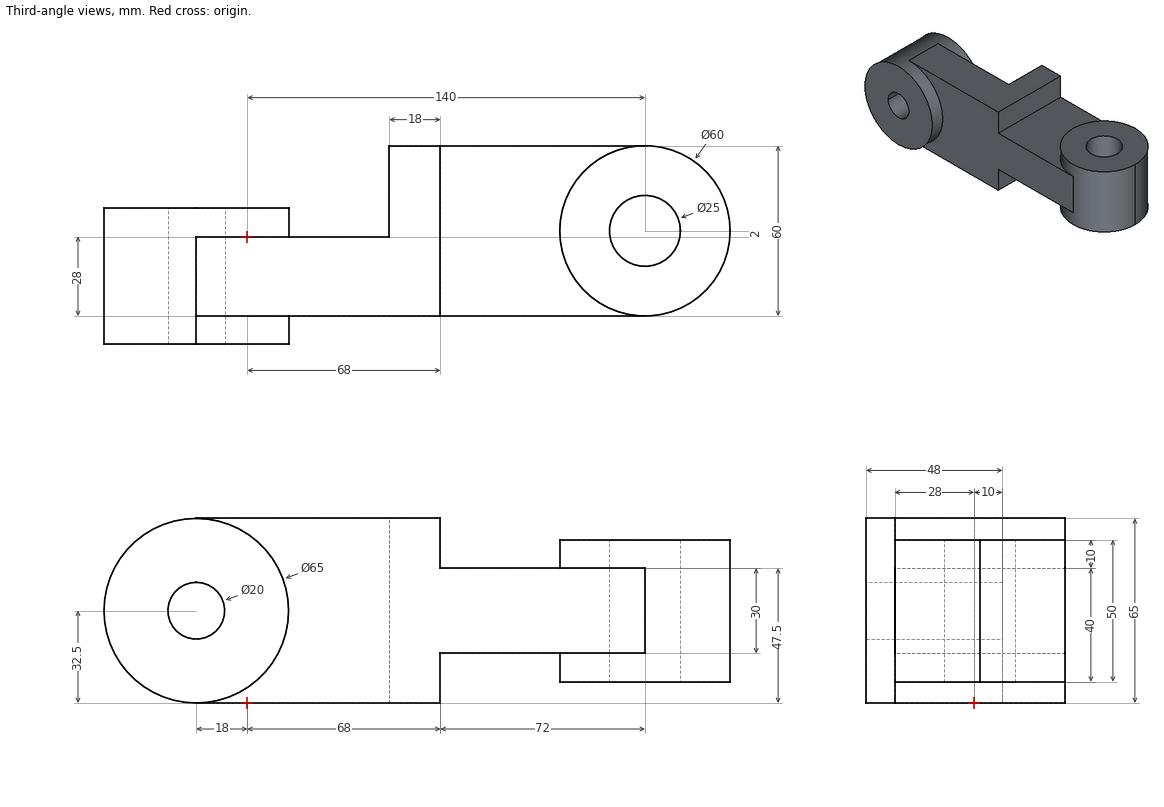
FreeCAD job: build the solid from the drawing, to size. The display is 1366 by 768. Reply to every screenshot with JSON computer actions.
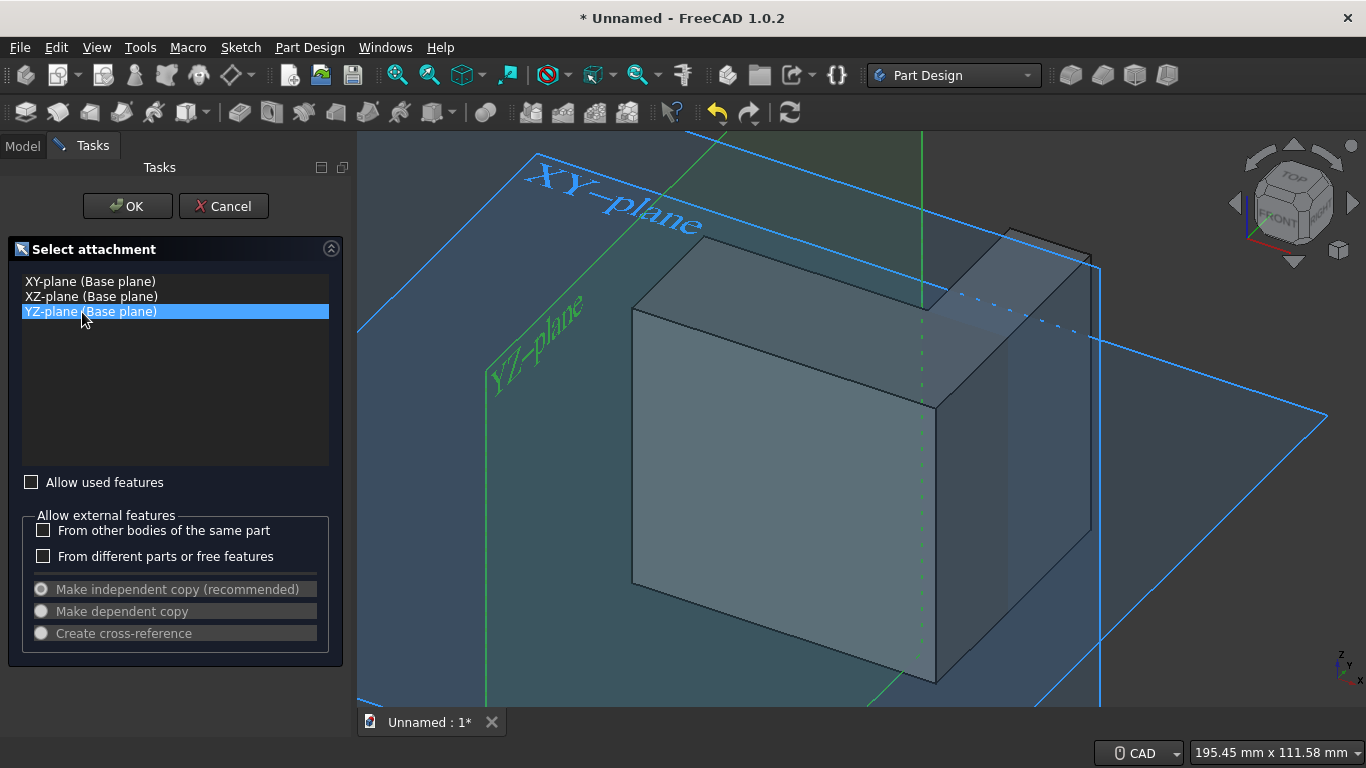
{"action": "left_click", "coordinate": [128, 206]}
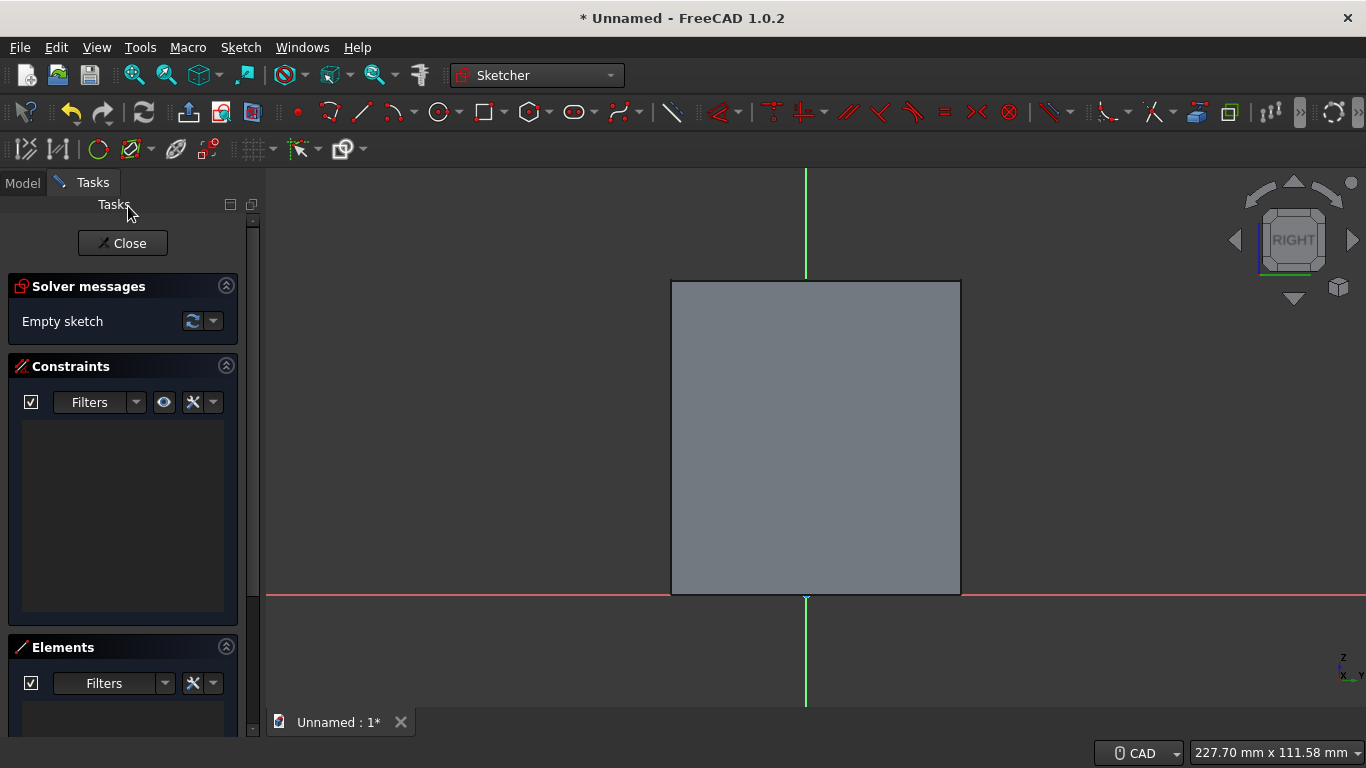
{"action": "key", "text": "q s"}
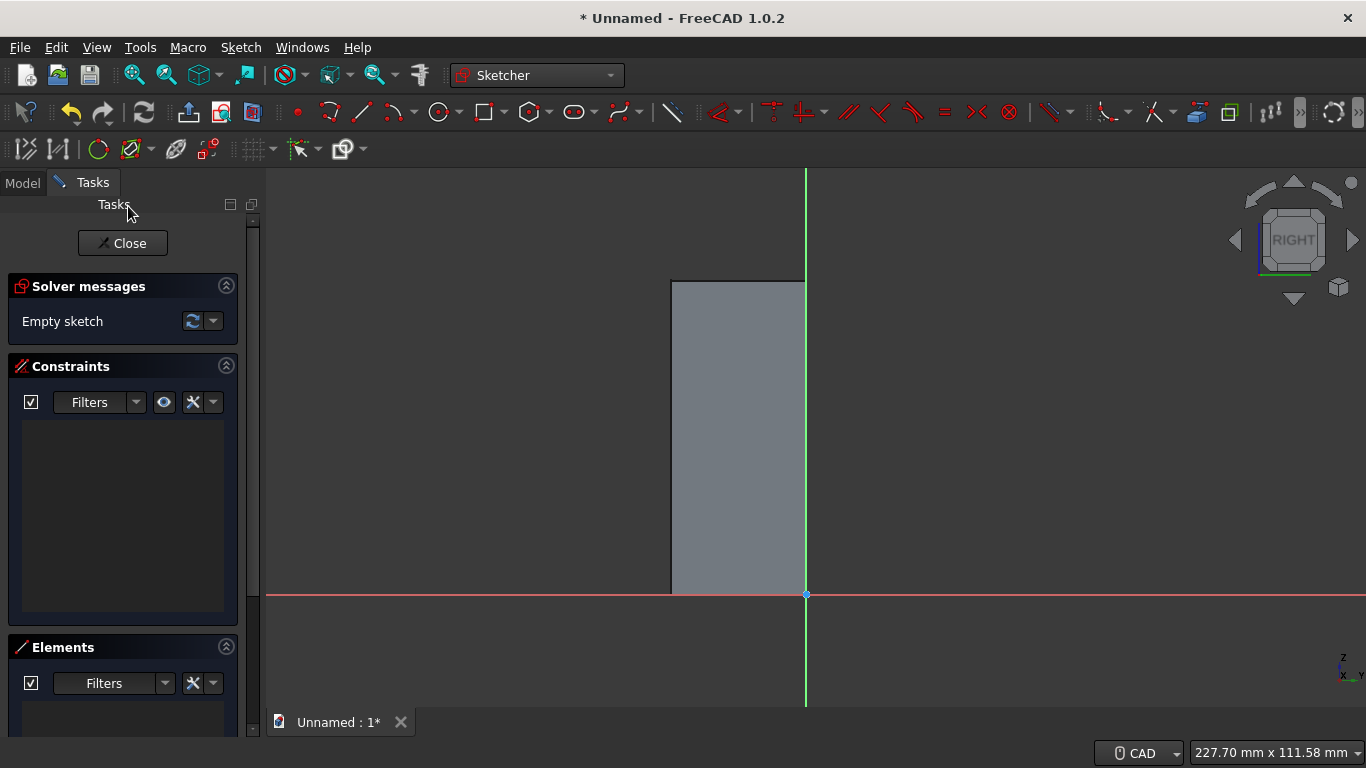
{"action": "key", "text": "g r"}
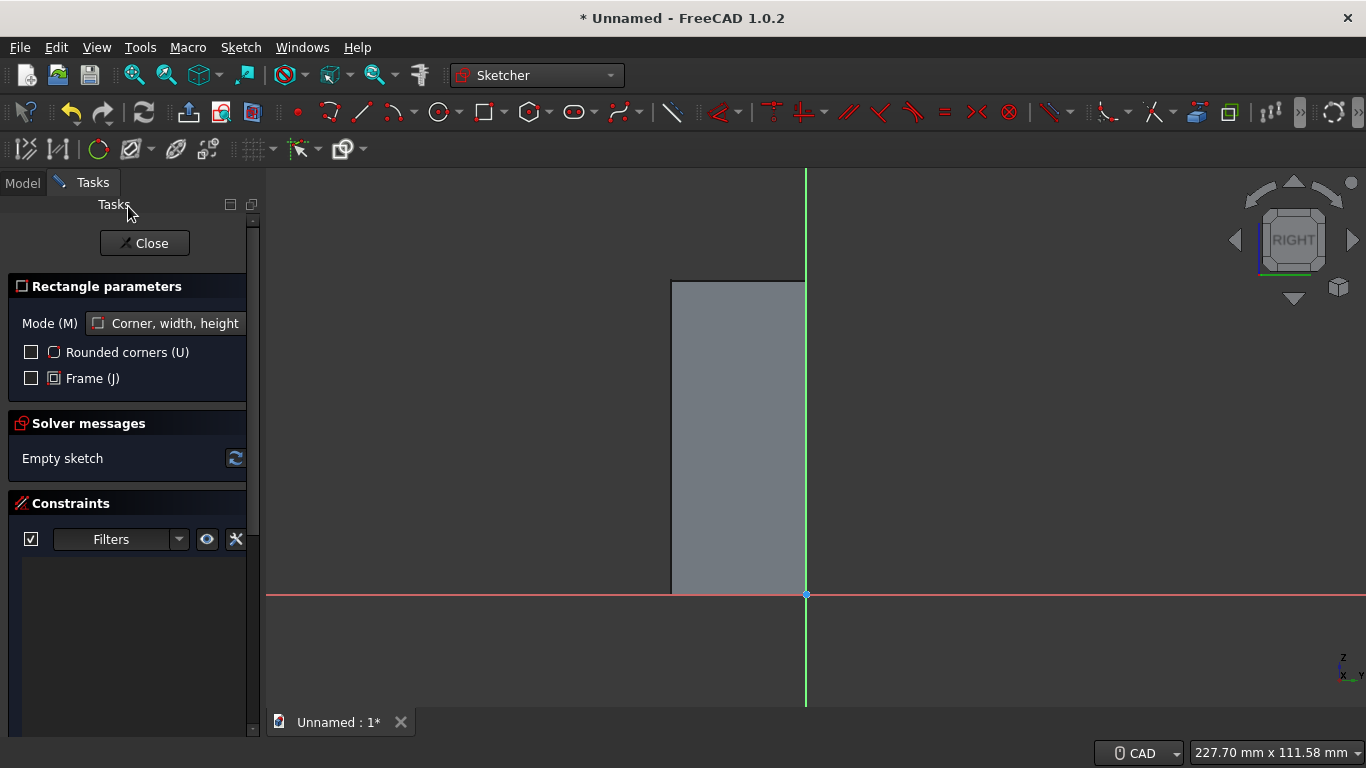
{"action": "left_click", "coordinate": [806, 595]}
{"action": "left_click", "coordinate": [671, 280]}
{"action": "key", "text": "Escape"}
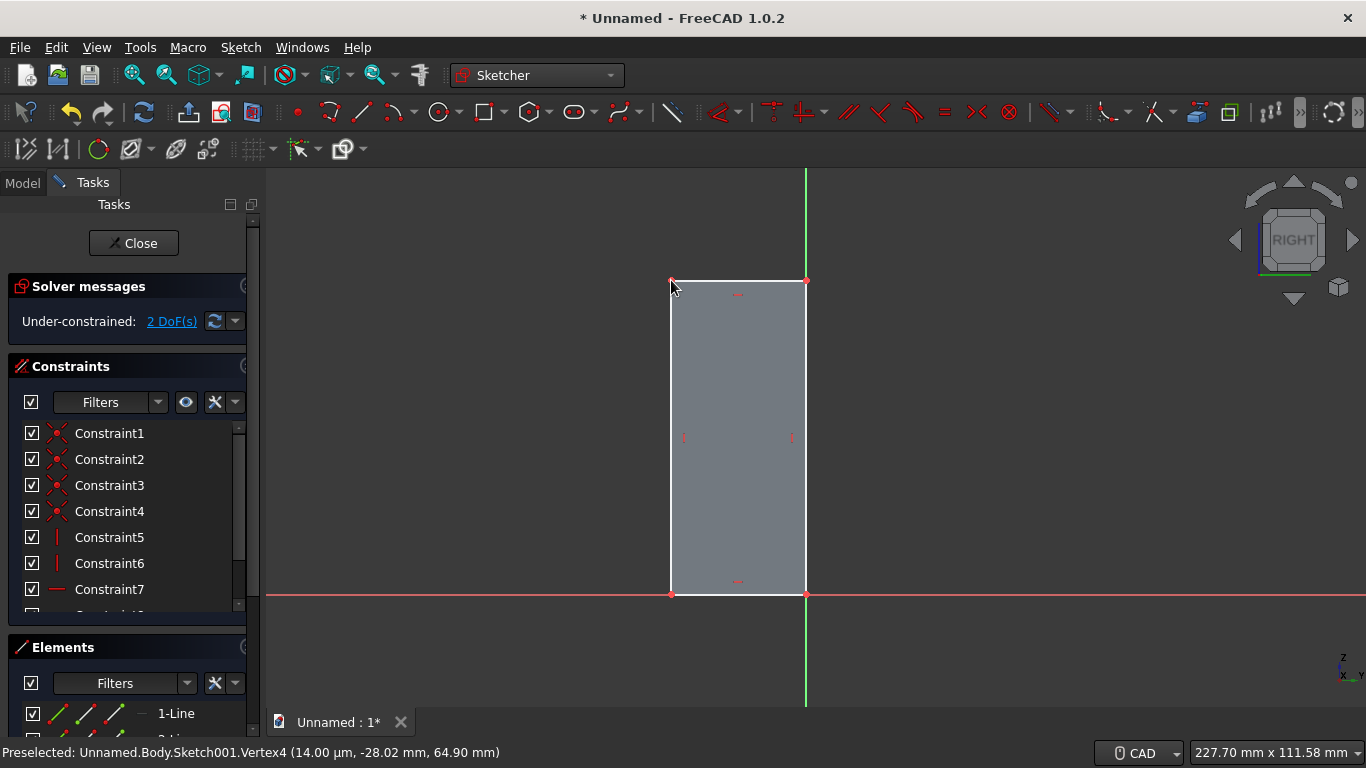
{"action": "key", "text": "d"}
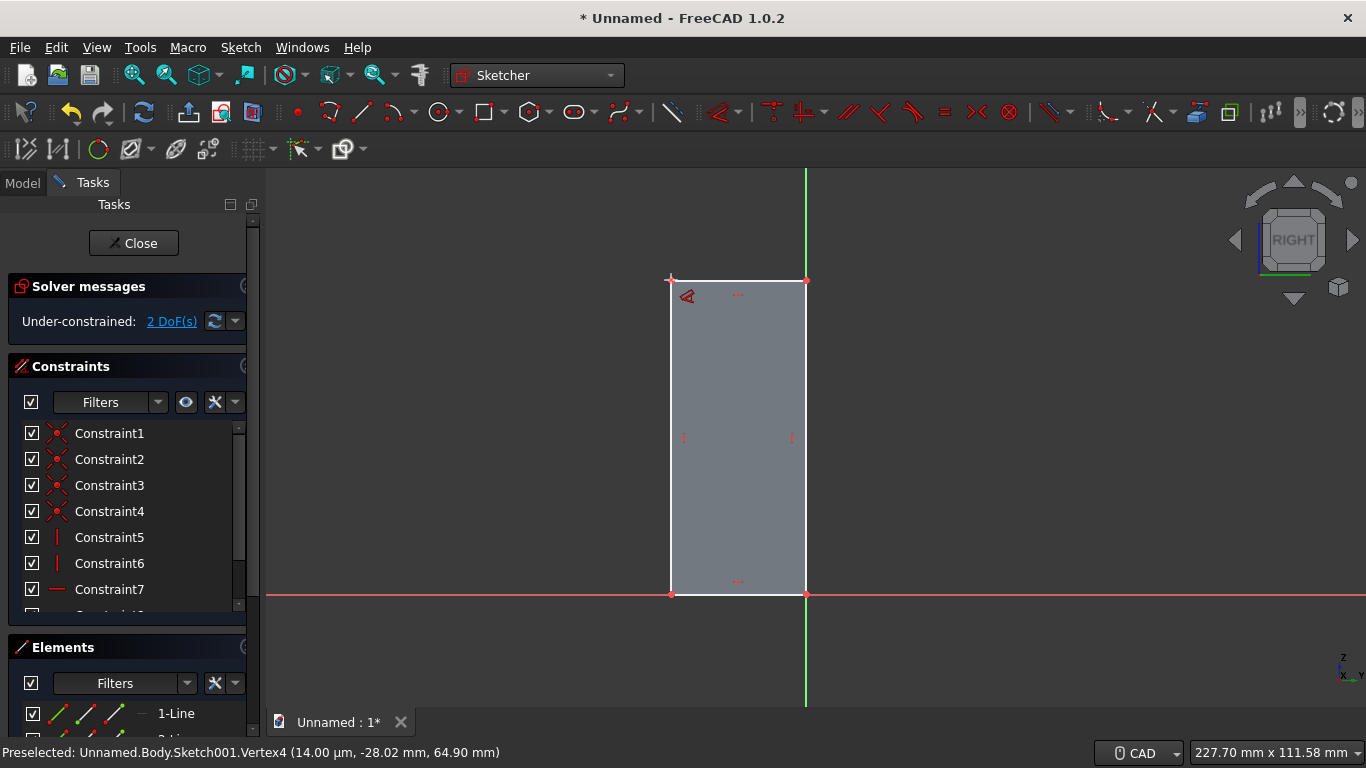
{"action": "left_click", "coordinate": [806, 500]}
{"action": "left_click", "coordinate": [840, 438]}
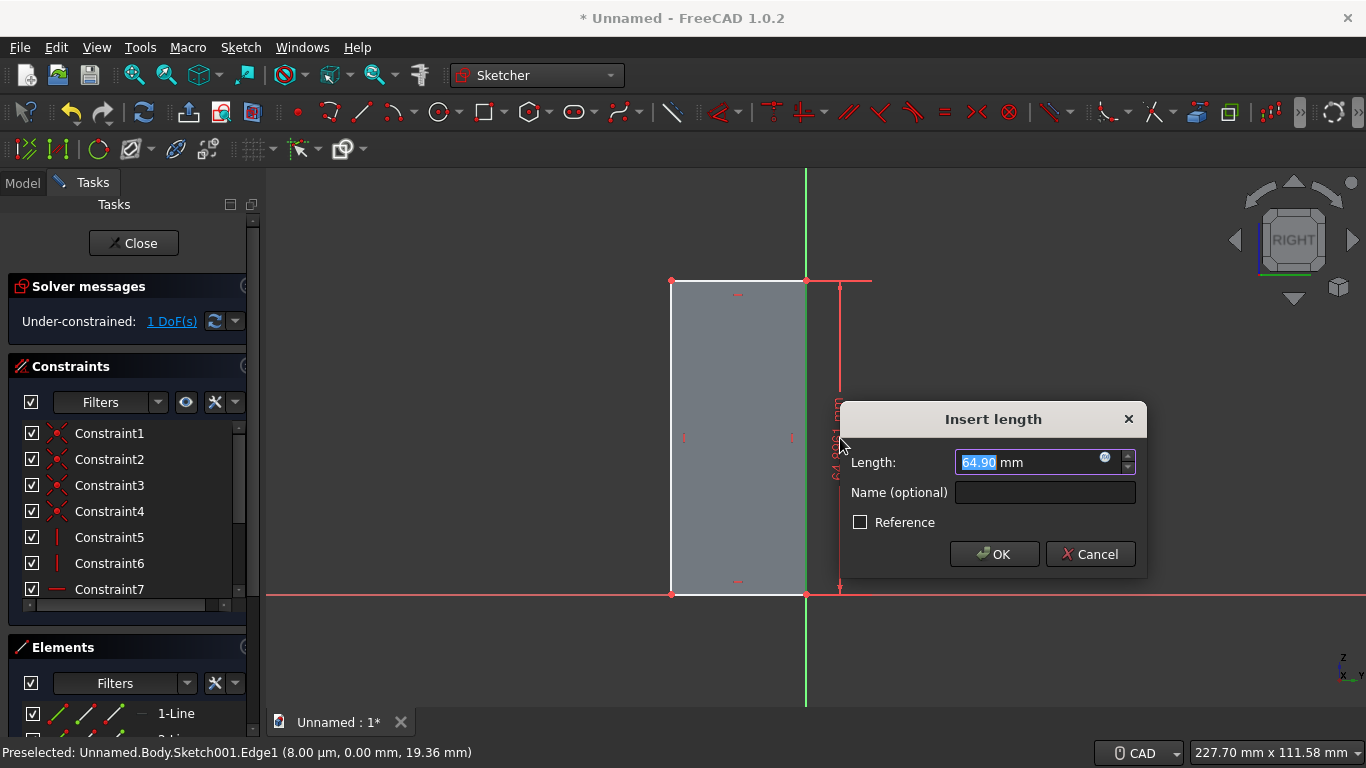
{"action": "type", "text": "65"}
{"action": "key", "text": "Return"}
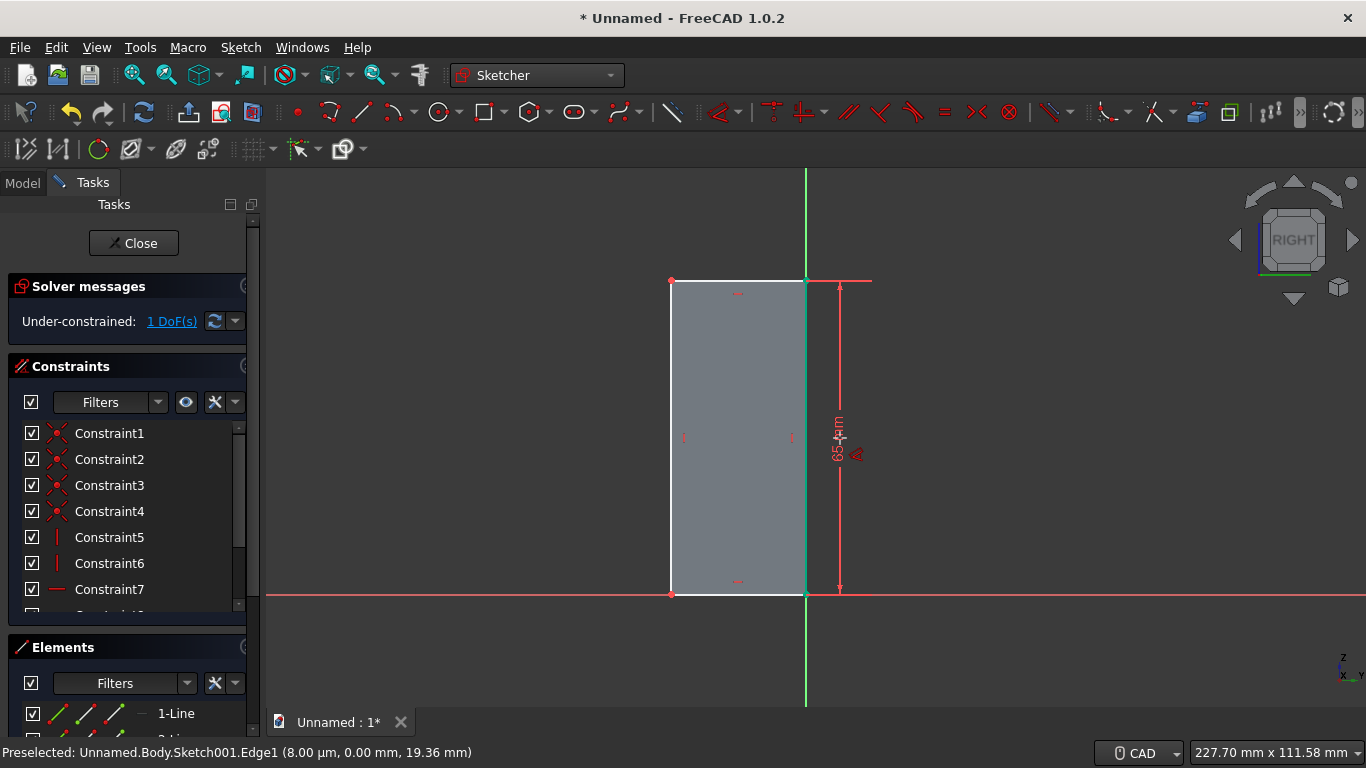
{"action": "left_click", "coordinate": [766, 280]}
{"action": "left_click", "coordinate": [739, 246]}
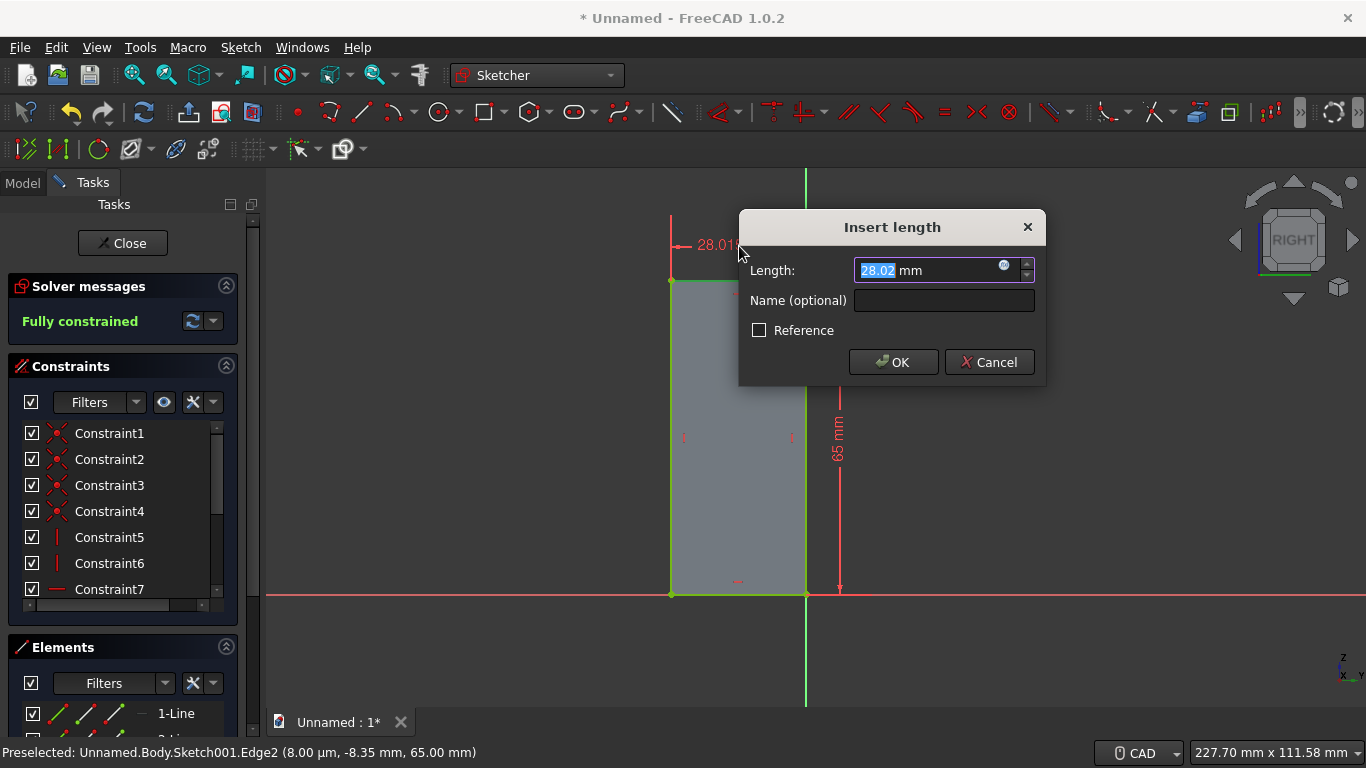
{"action": "type", "text": "28"}
{"action": "key", "text": "Return"}
{"action": "key", "text": "Escape"}